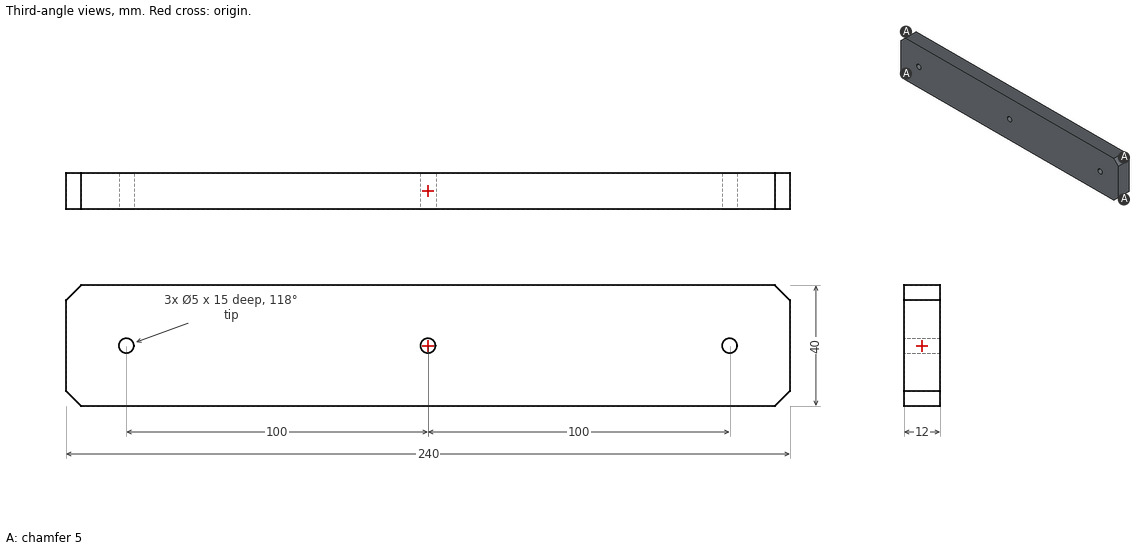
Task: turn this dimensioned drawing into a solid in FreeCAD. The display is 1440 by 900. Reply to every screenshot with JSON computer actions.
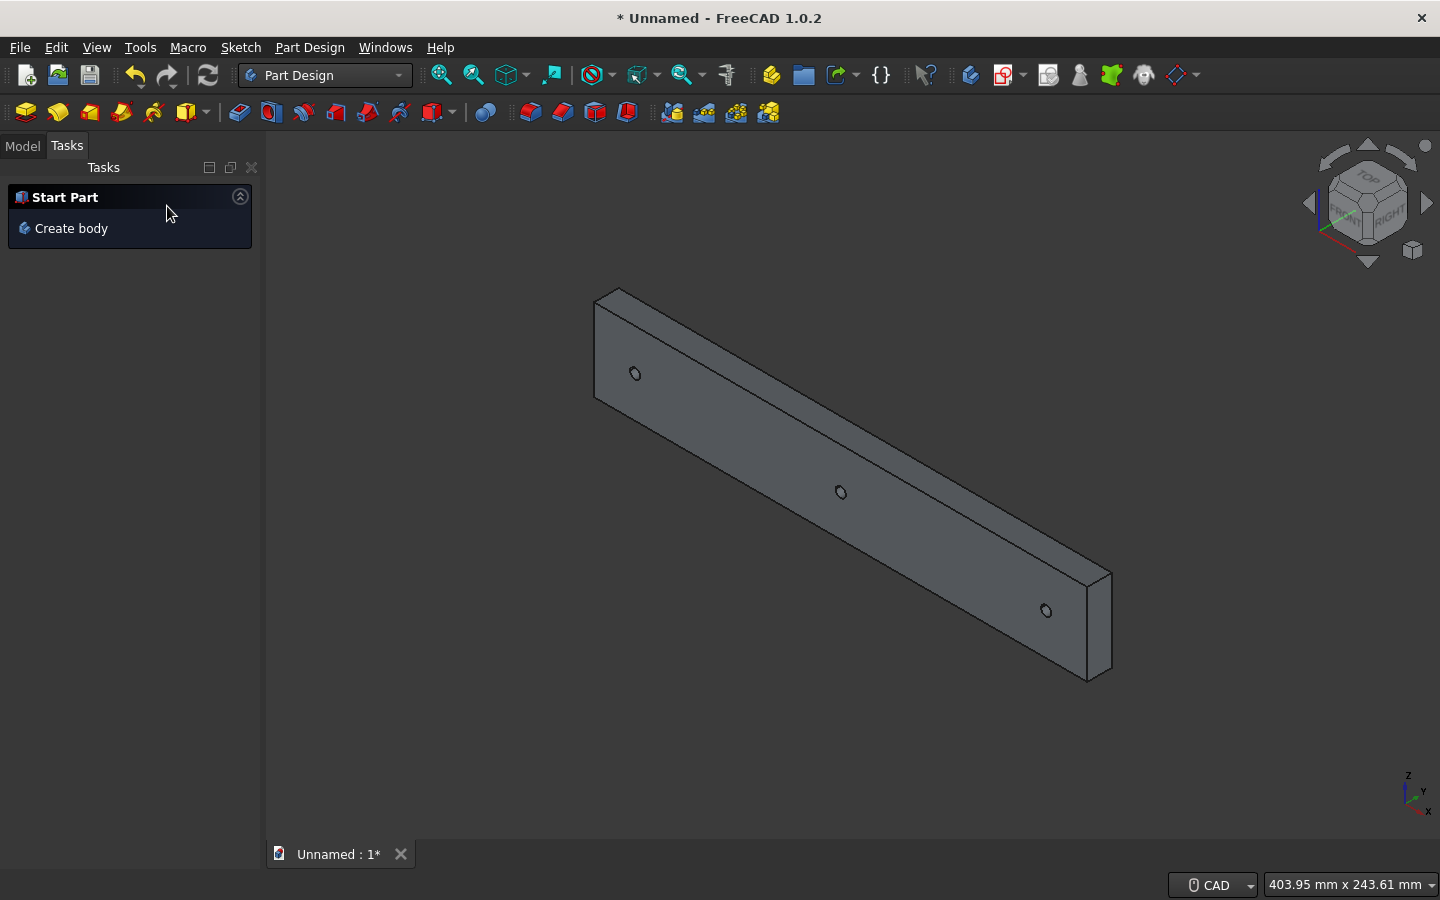
{"action": "left_click", "coordinate": [1100, 579]}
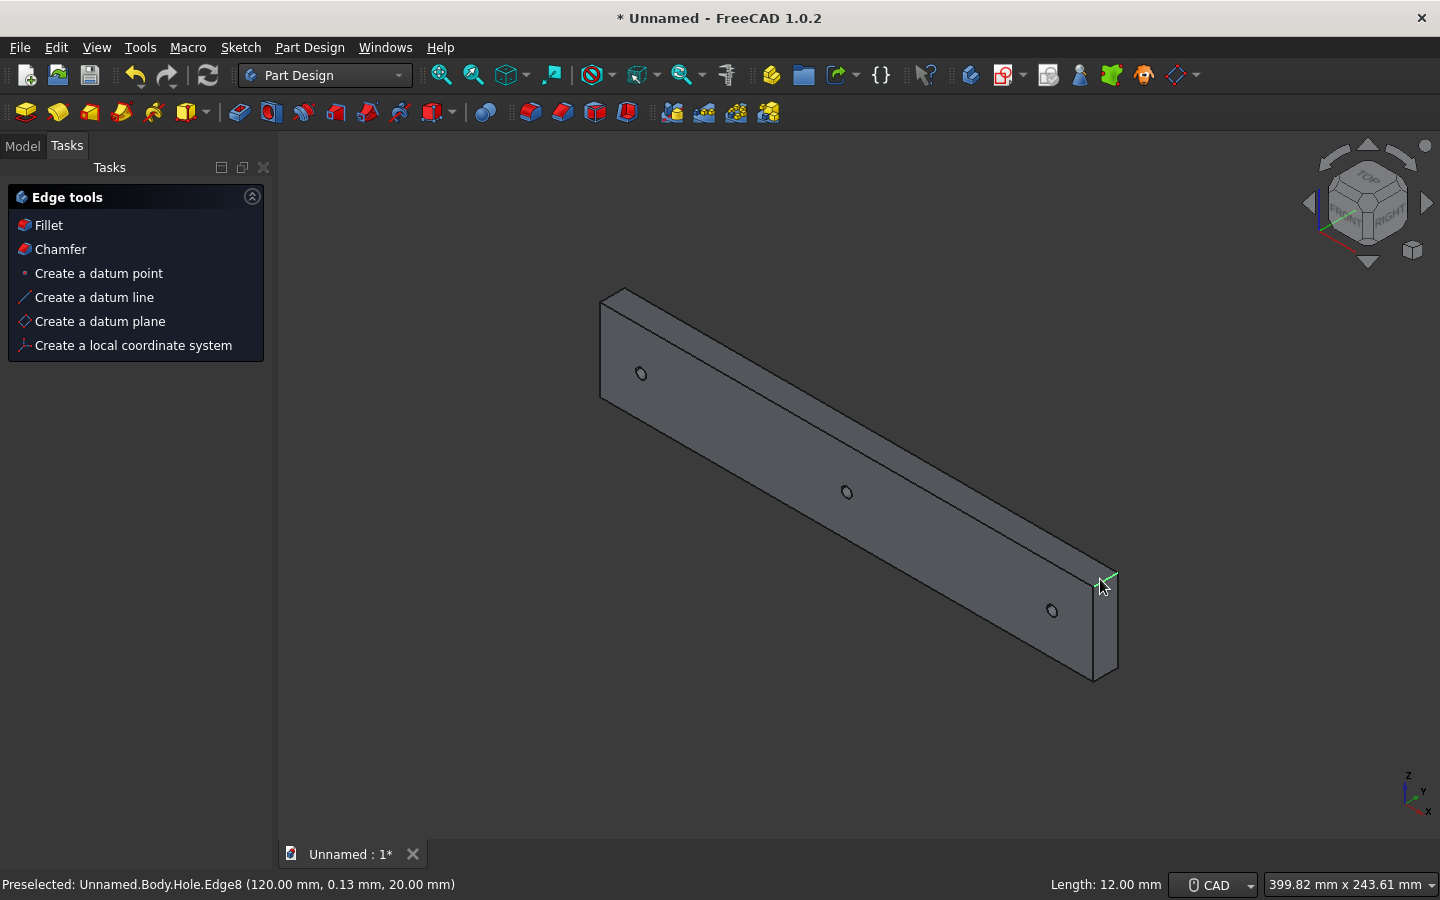
{"action": "key", "text": "2"}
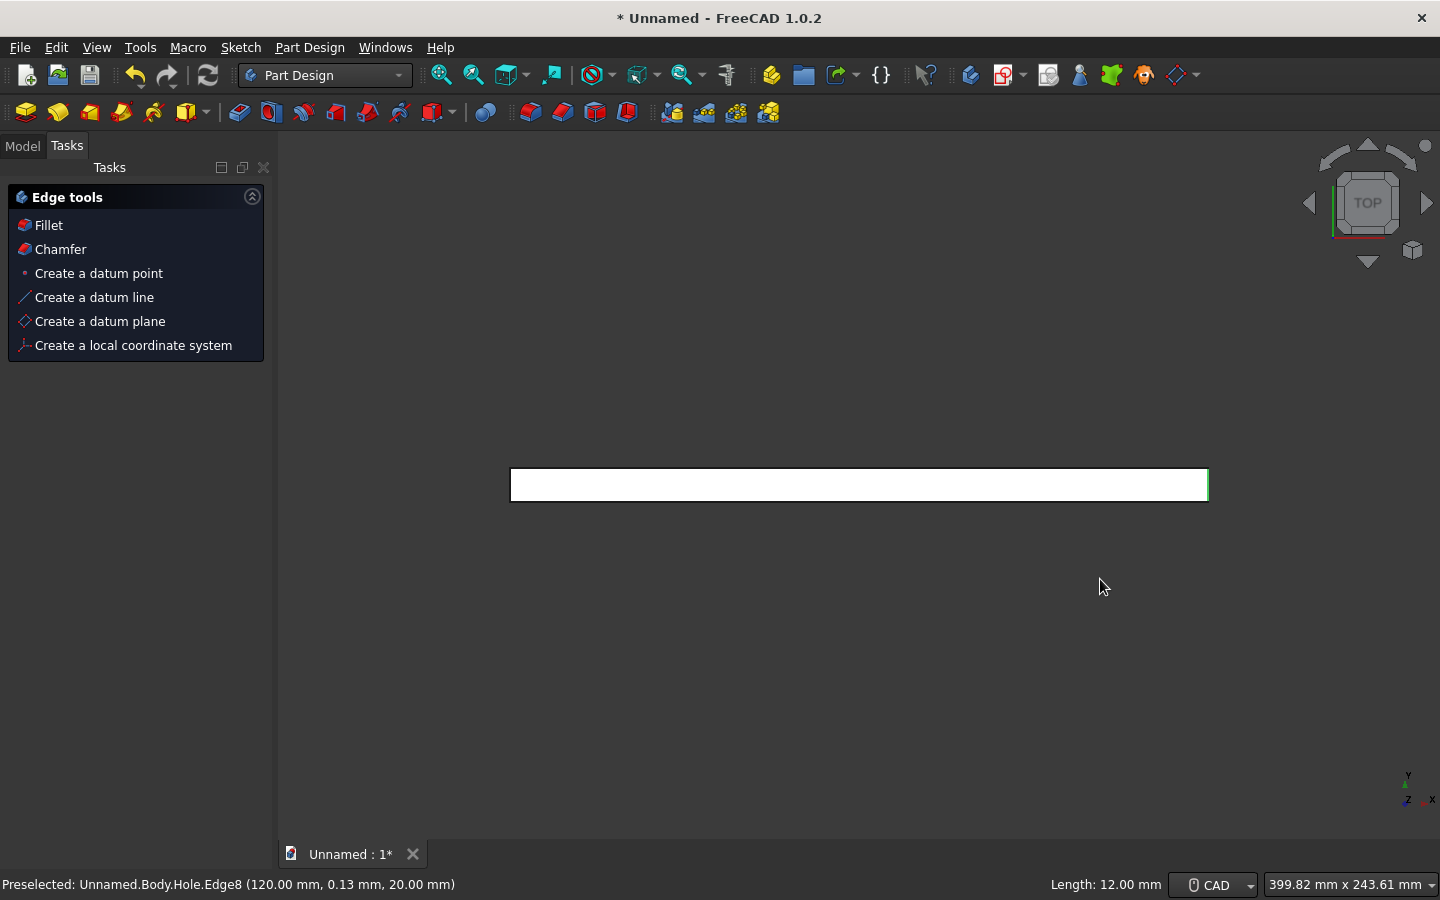
{"action": "left_click", "coordinate": [510, 484], "text": "ctrl"}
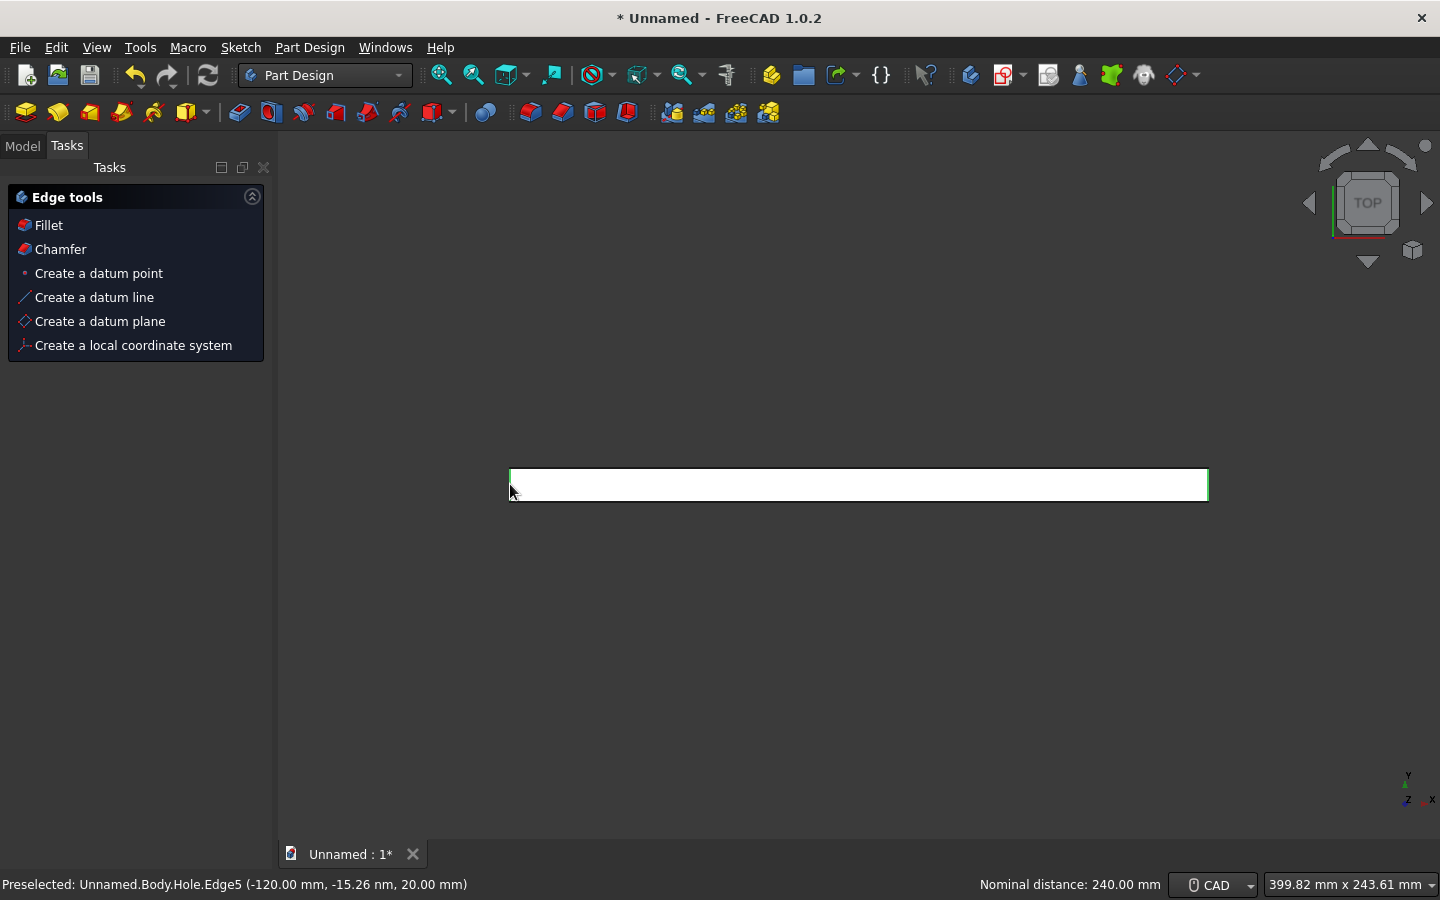
{"action": "key", "text": "1"}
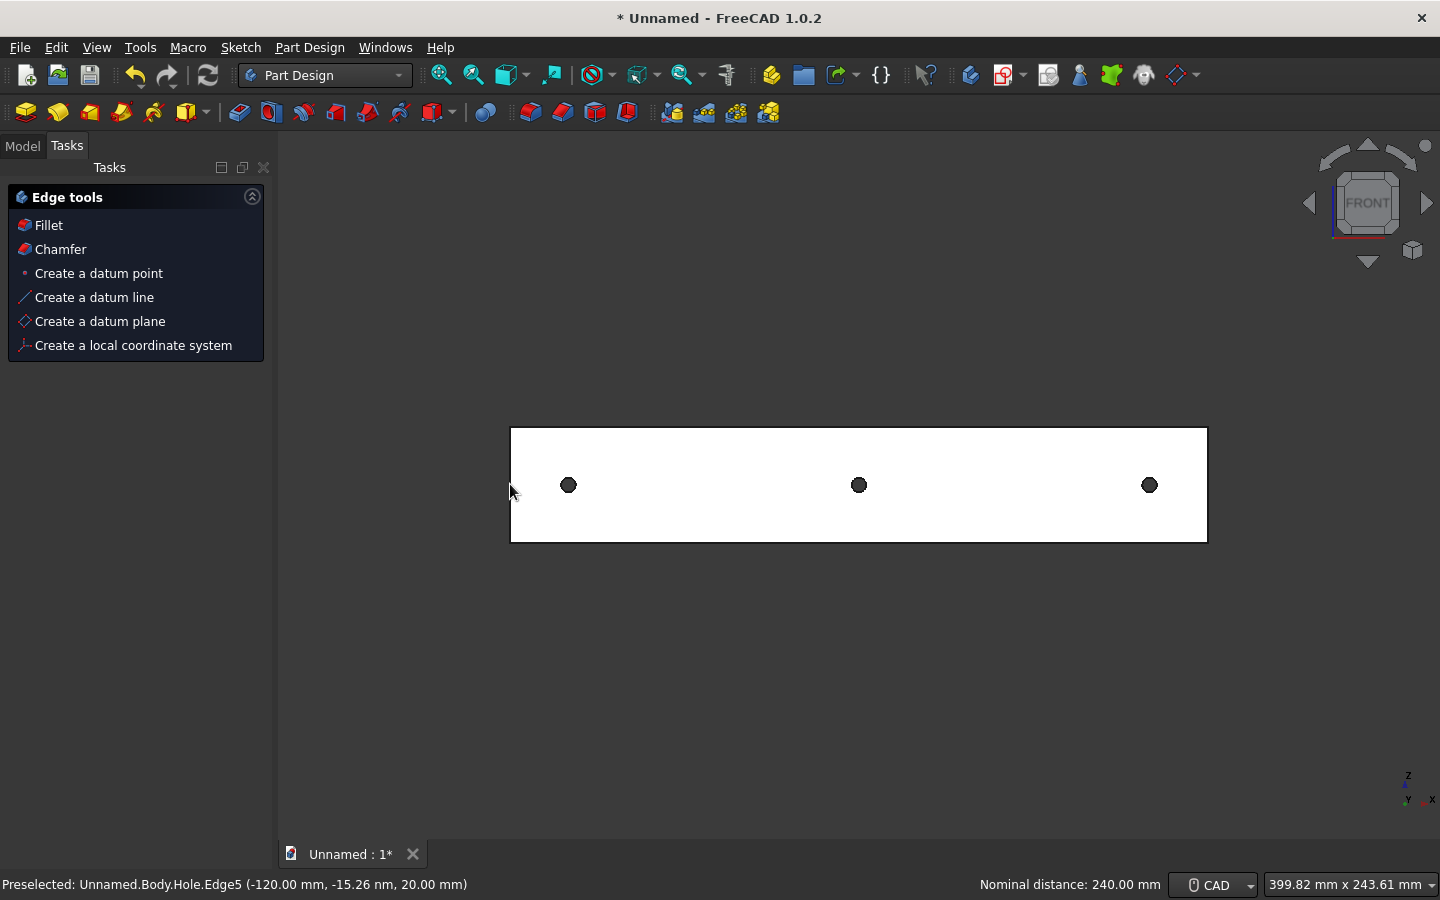
{"action": "key", "text": "3"}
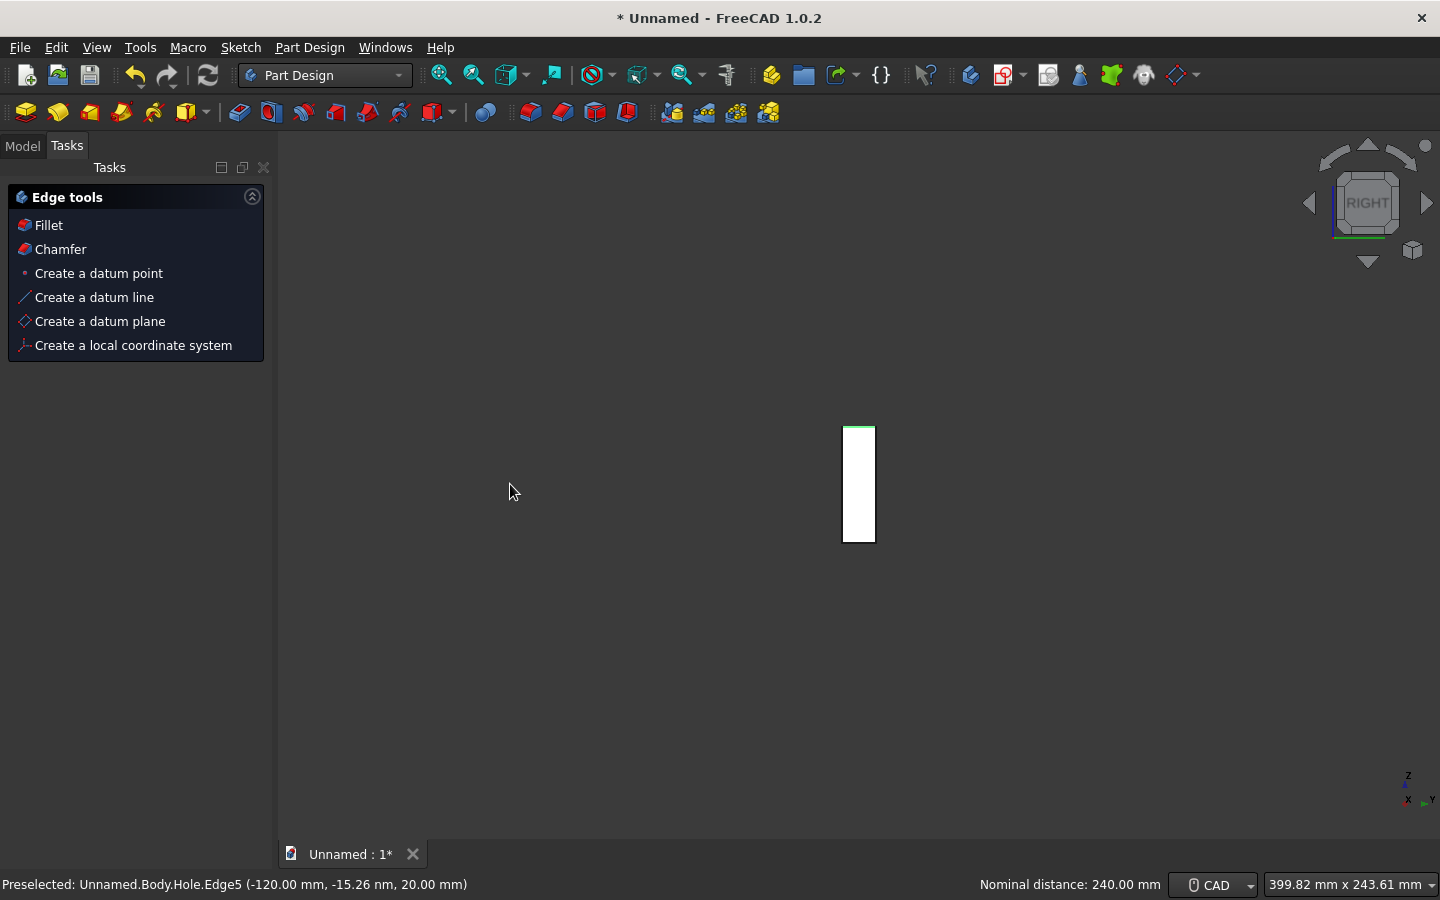
{"action": "left_click", "coordinate": [442, 76]}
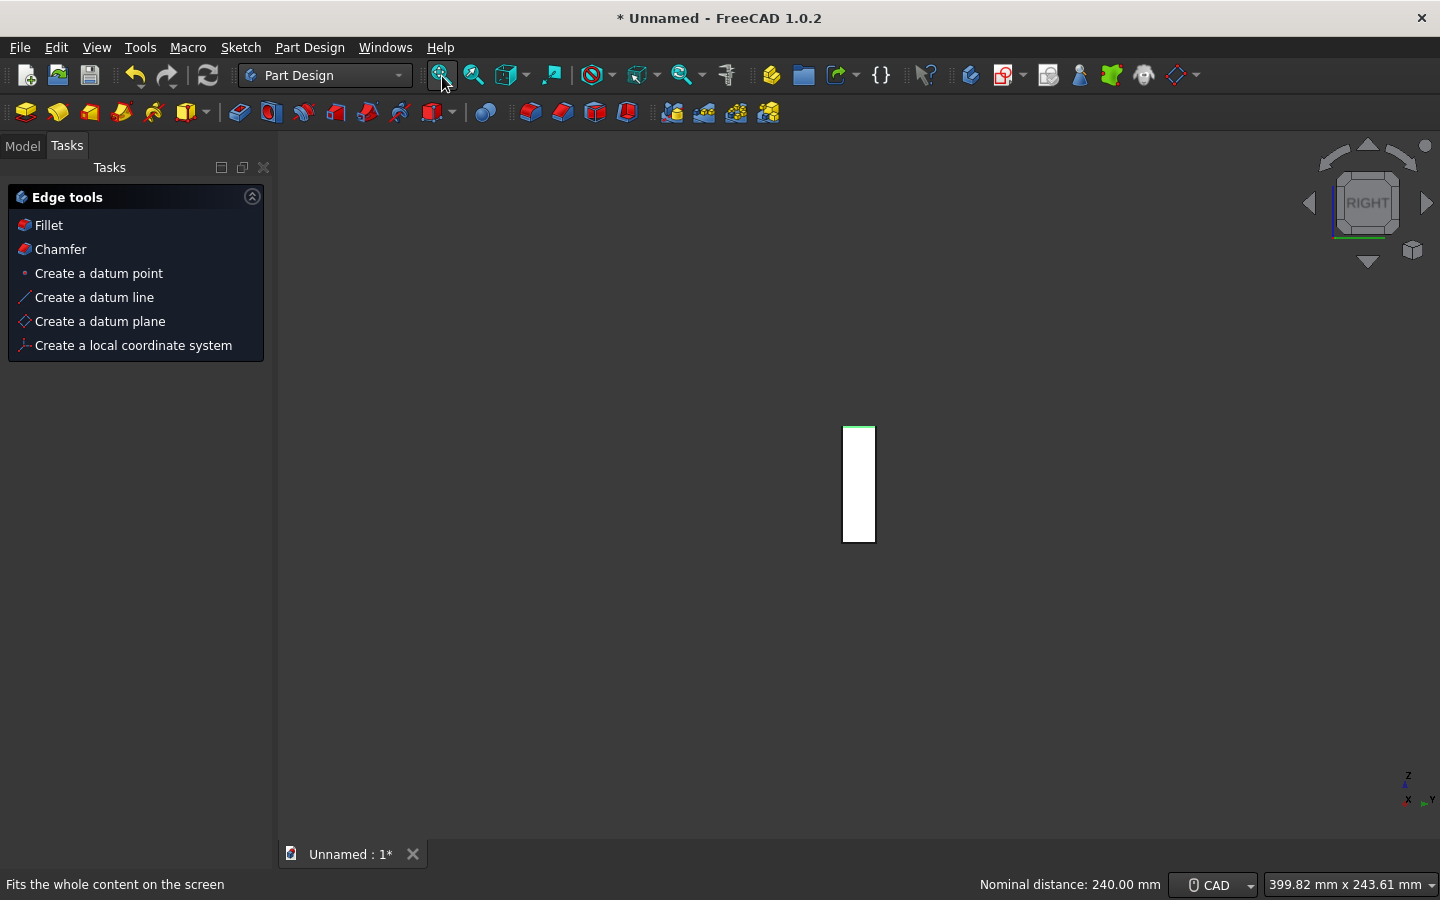
{"action": "left_click", "coordinate": [859, 542], "text": "ctrl"}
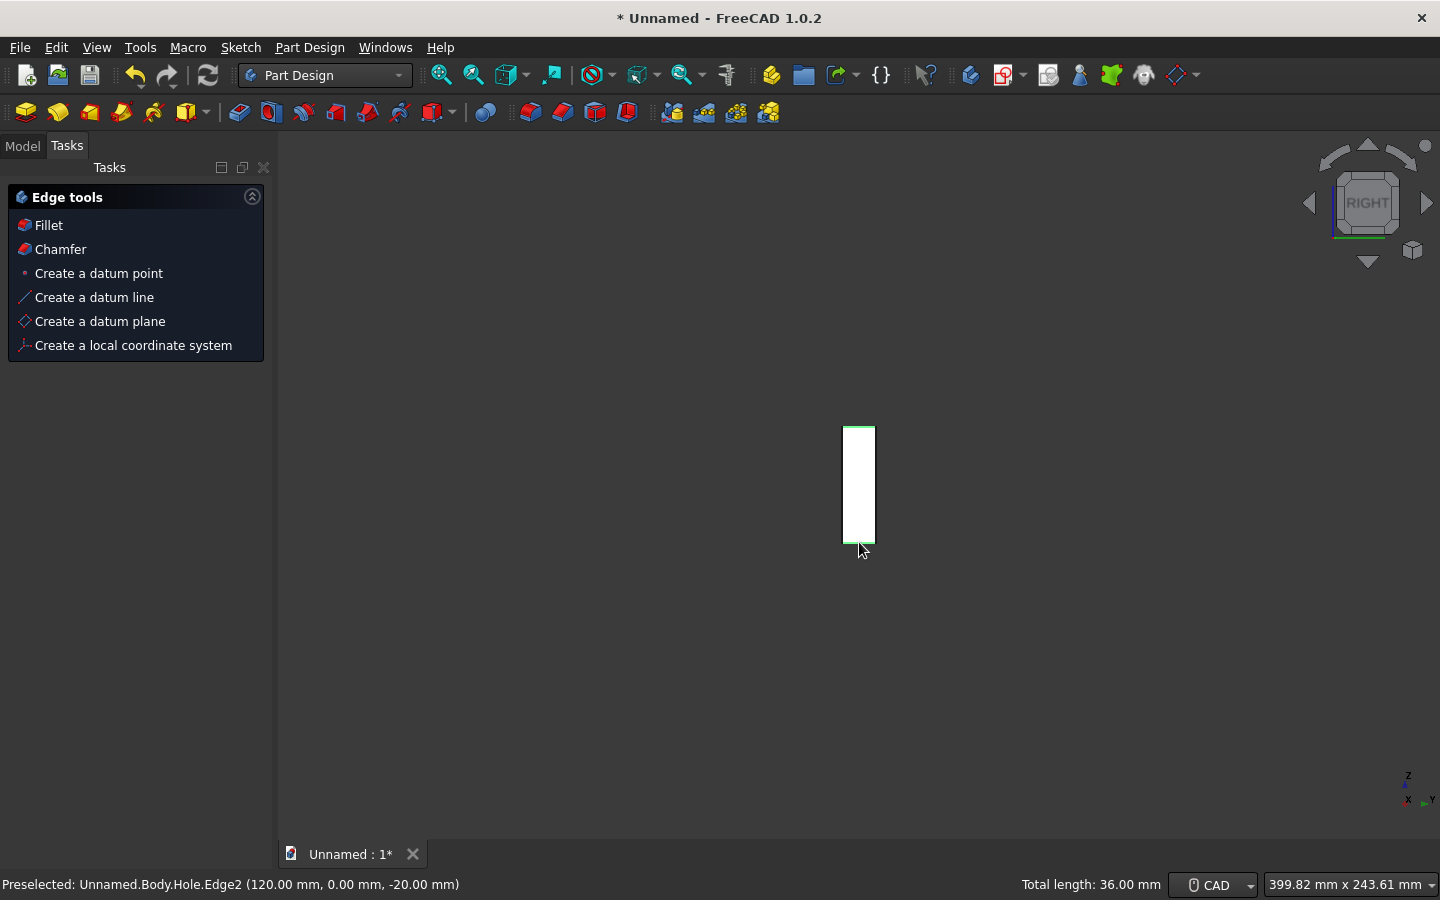
{"action": "key", "text": "5"}